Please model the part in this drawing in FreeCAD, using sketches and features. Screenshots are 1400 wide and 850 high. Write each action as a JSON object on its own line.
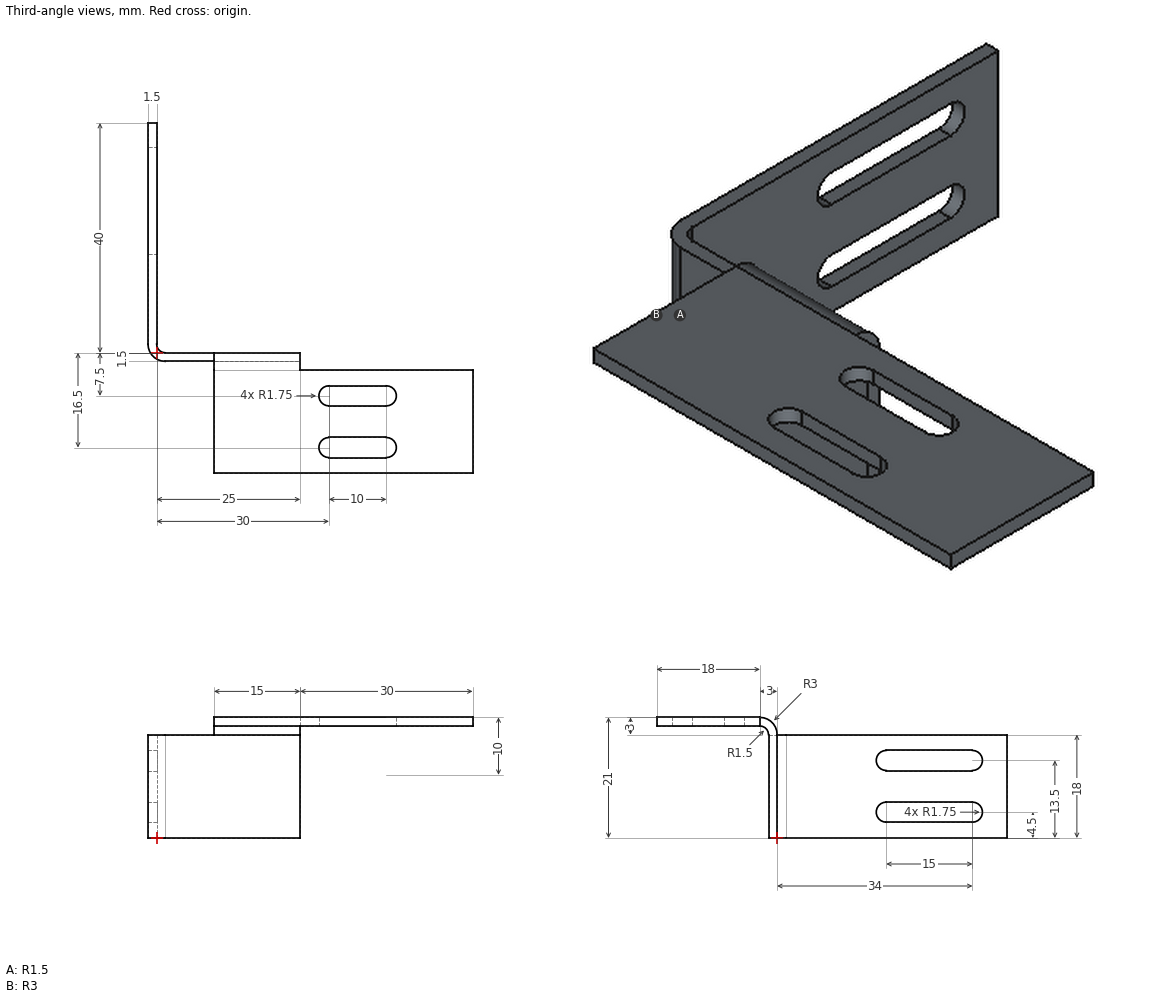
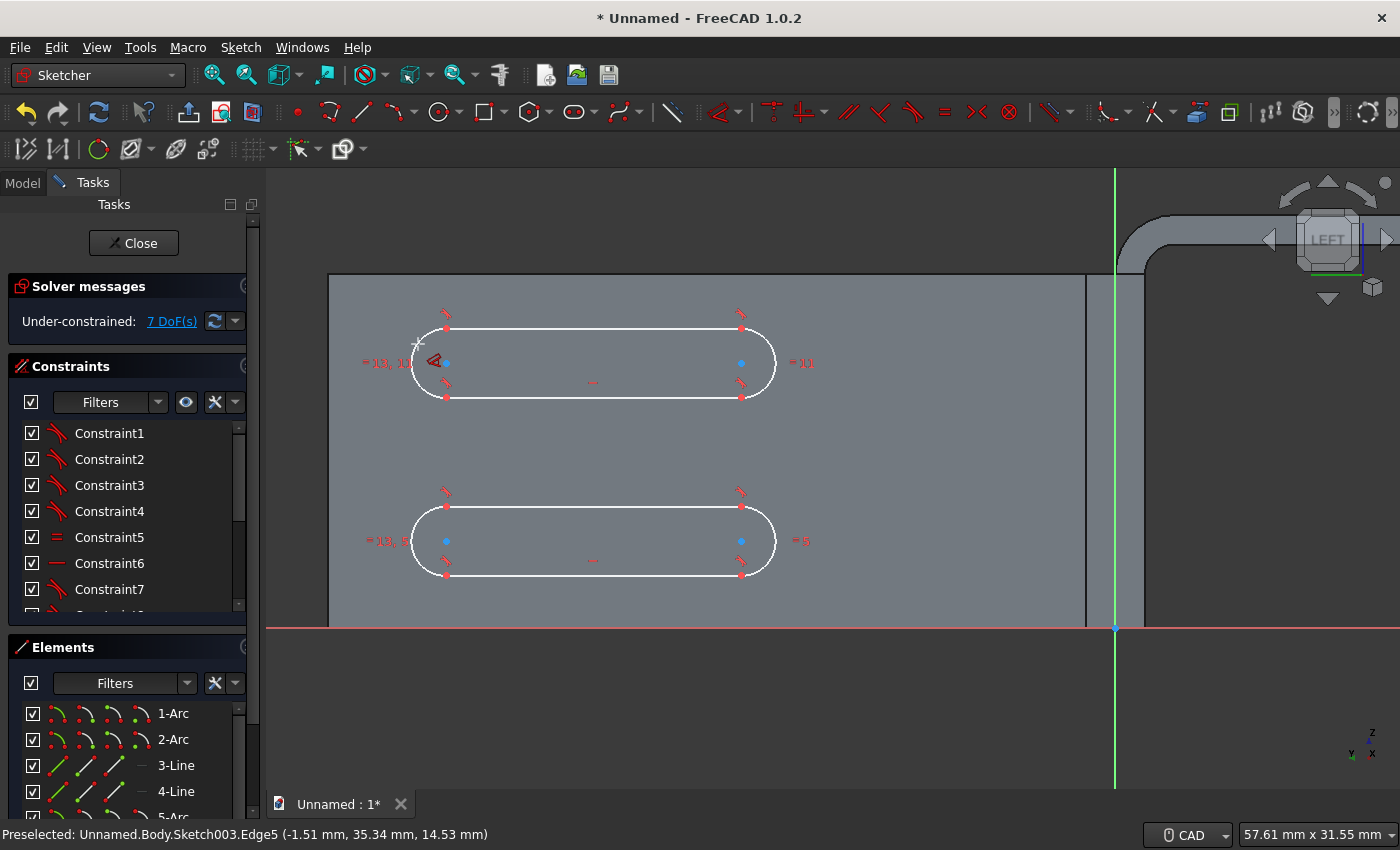
{"action": "left_click", "coordinate": [418, 521]}
{"action": "left_click", "coordinate": [392, 502]}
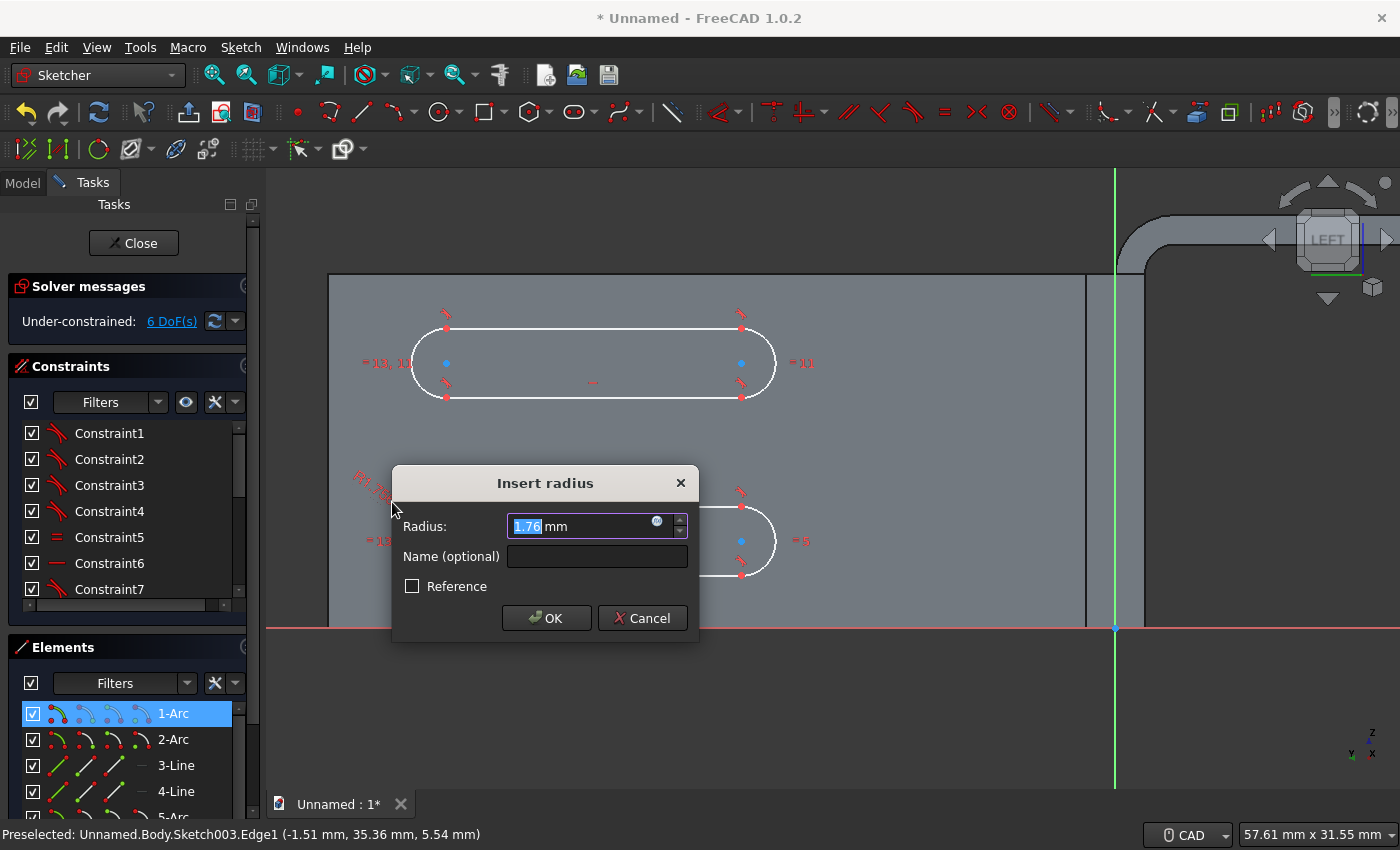
{"action": "type", "text": "1.75"}
{"action": "key", "text": "Return"}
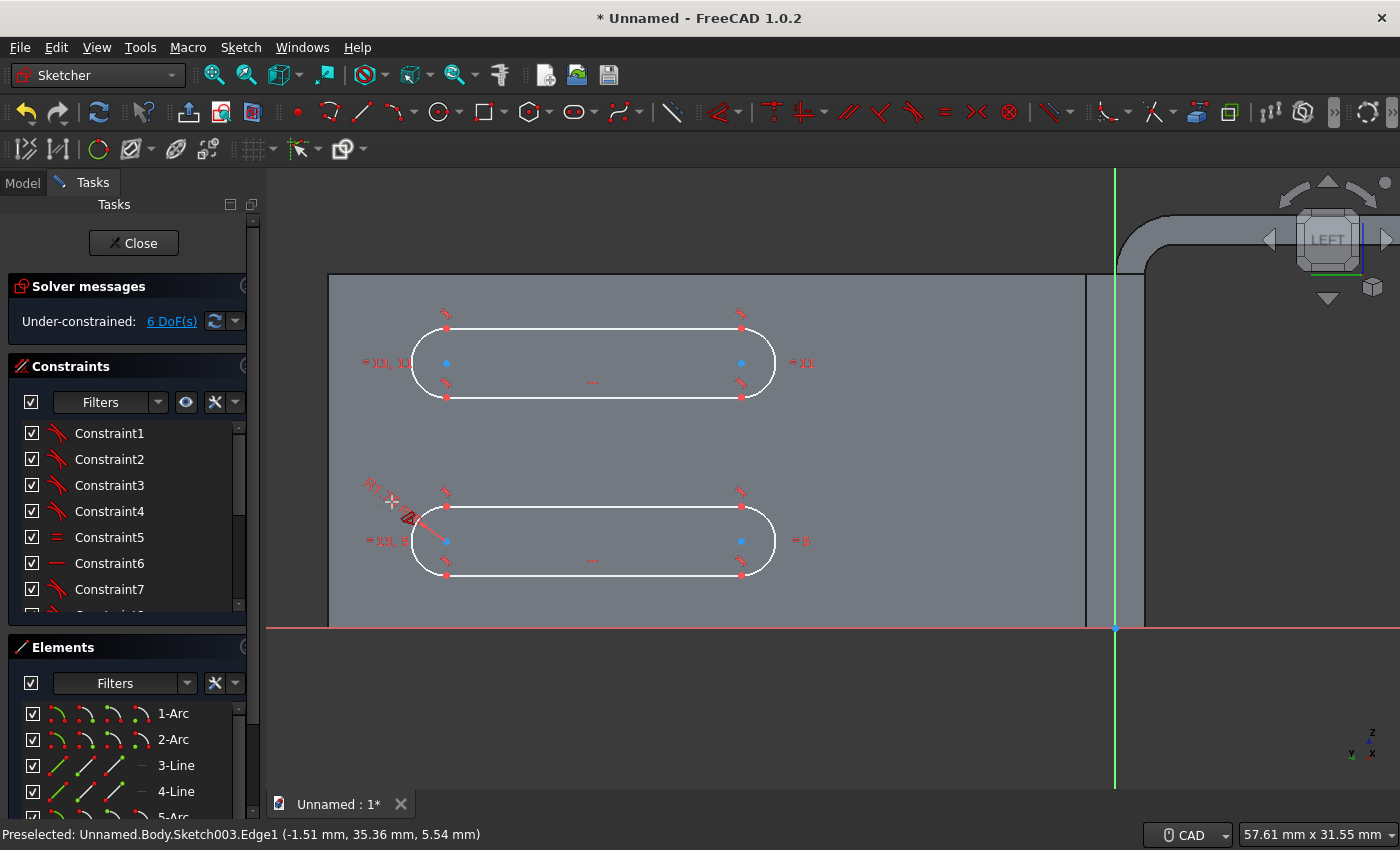
{"action": "left_click", "coordinate": [534, 507]}
{"action": "left_click", "coordinate": [594, 541]}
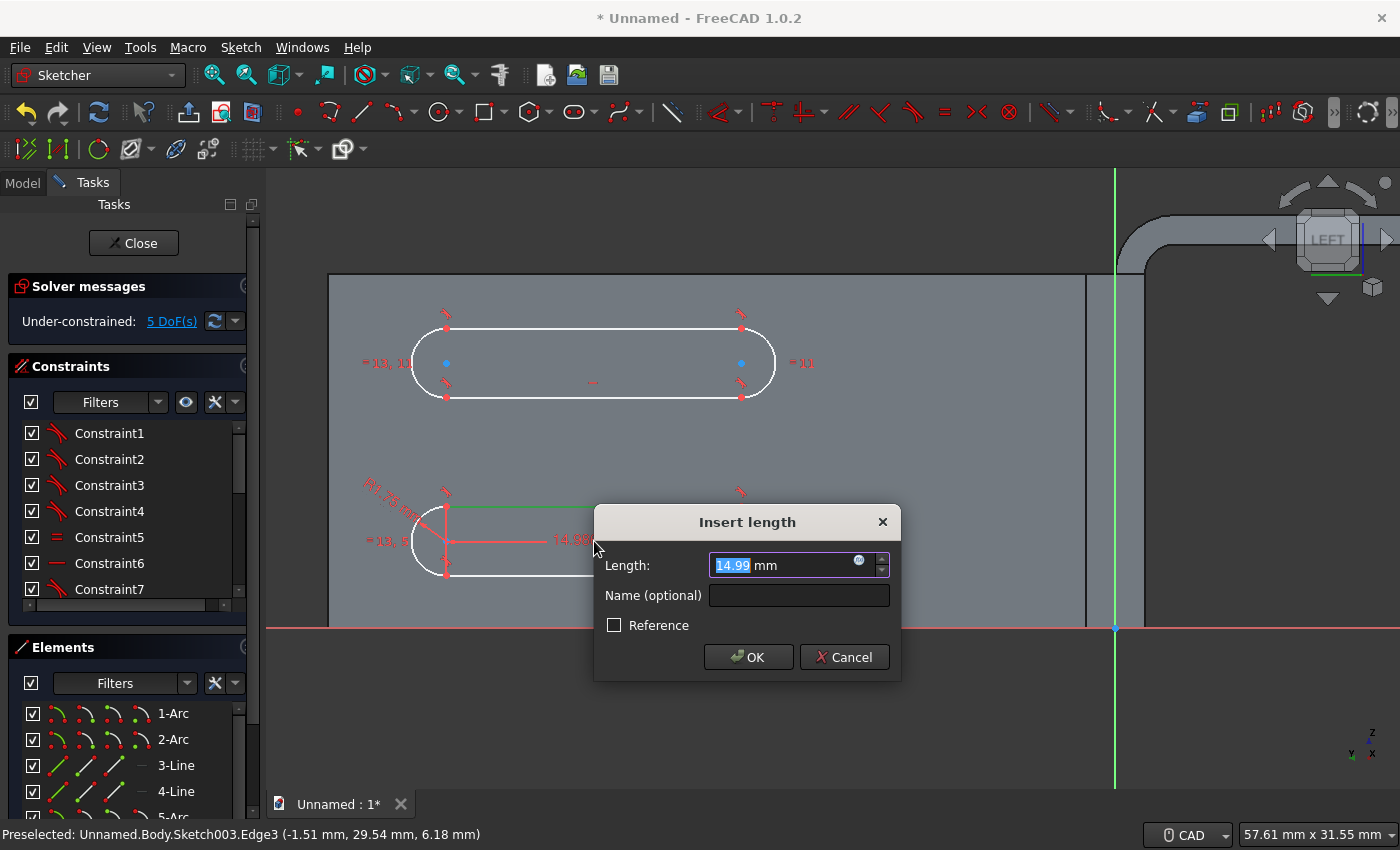
{"action": "type", "text": "15"}
{"action": "key", "text": "Return"}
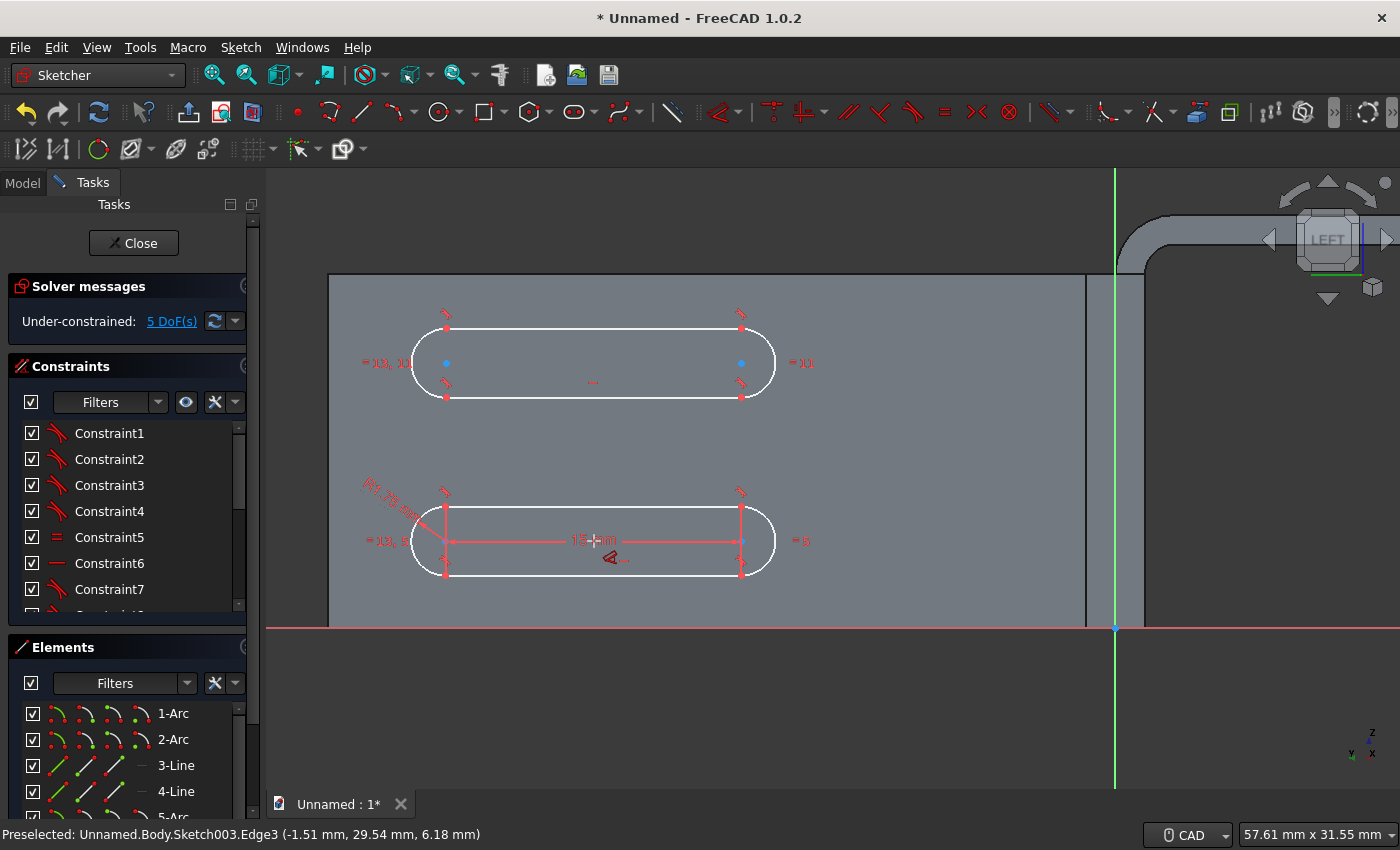
{"action": "left_click", "coordinate": [535, 329]}
{"action": "left_click", "coordinate": [594, 295]}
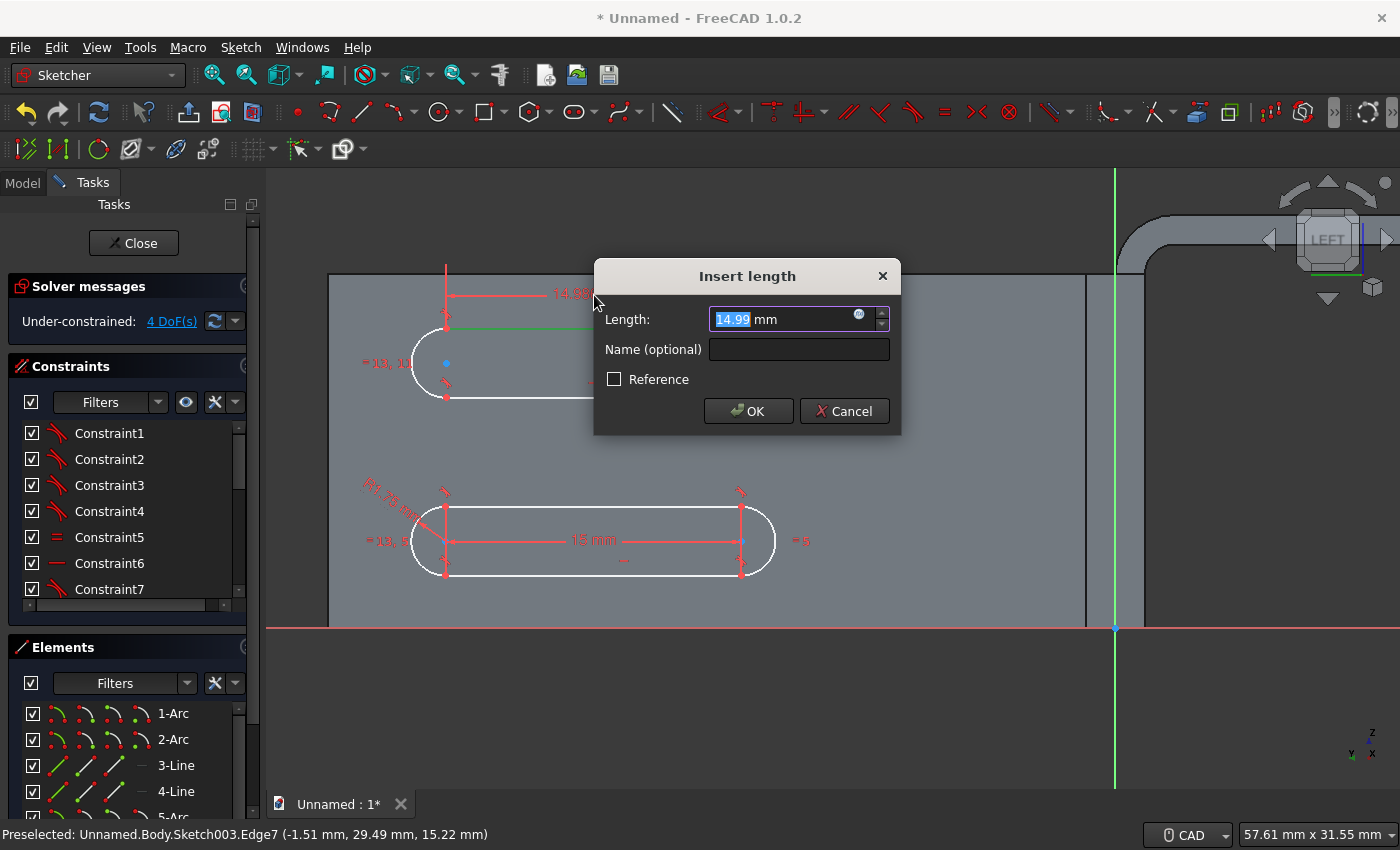
{"action": "type", "text": "15"}
{"action": "key", "text": "Return"}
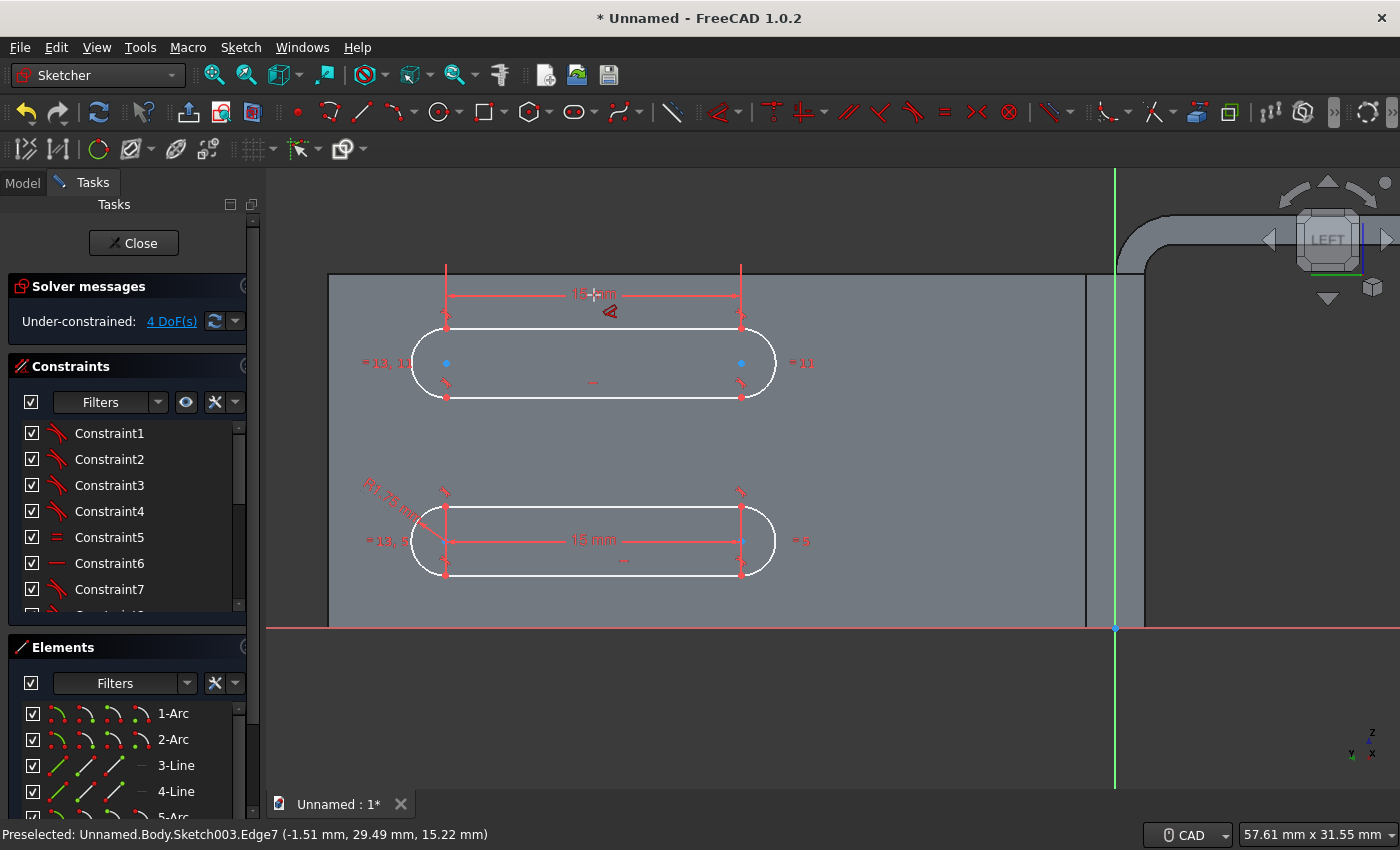
{"action": "left_click", "coordinate": [446, 507]}
{"action": "left_click", "coordinate": [781, 662]}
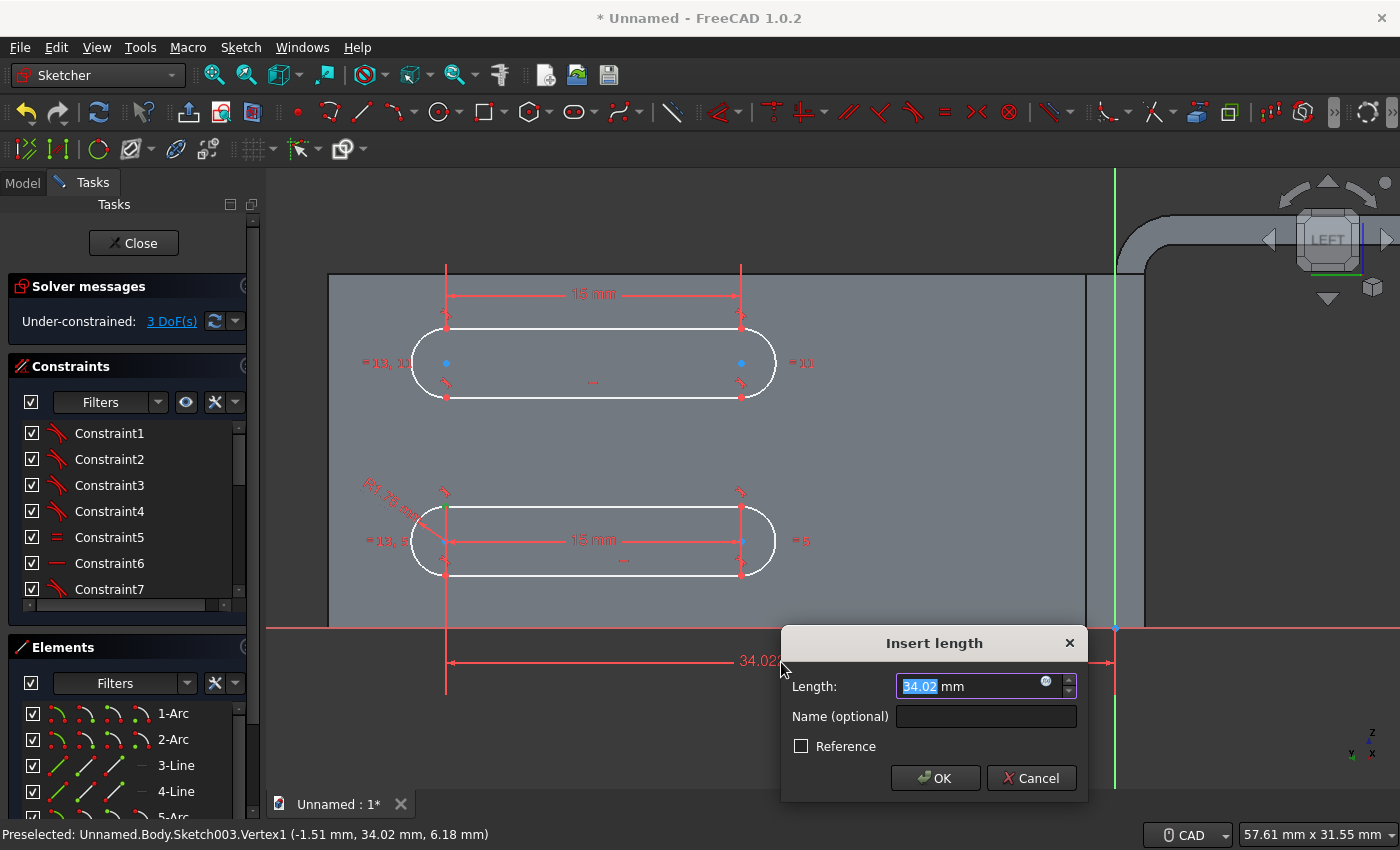
{"action": "type", "text": "34"}
{"action": "key", "text": "Return"}